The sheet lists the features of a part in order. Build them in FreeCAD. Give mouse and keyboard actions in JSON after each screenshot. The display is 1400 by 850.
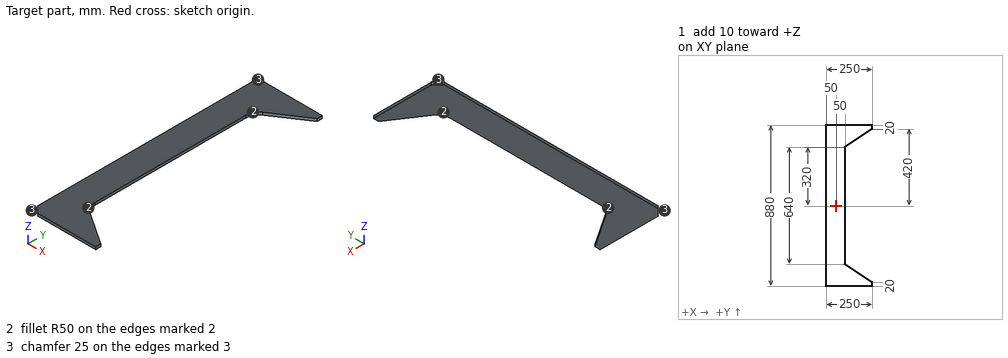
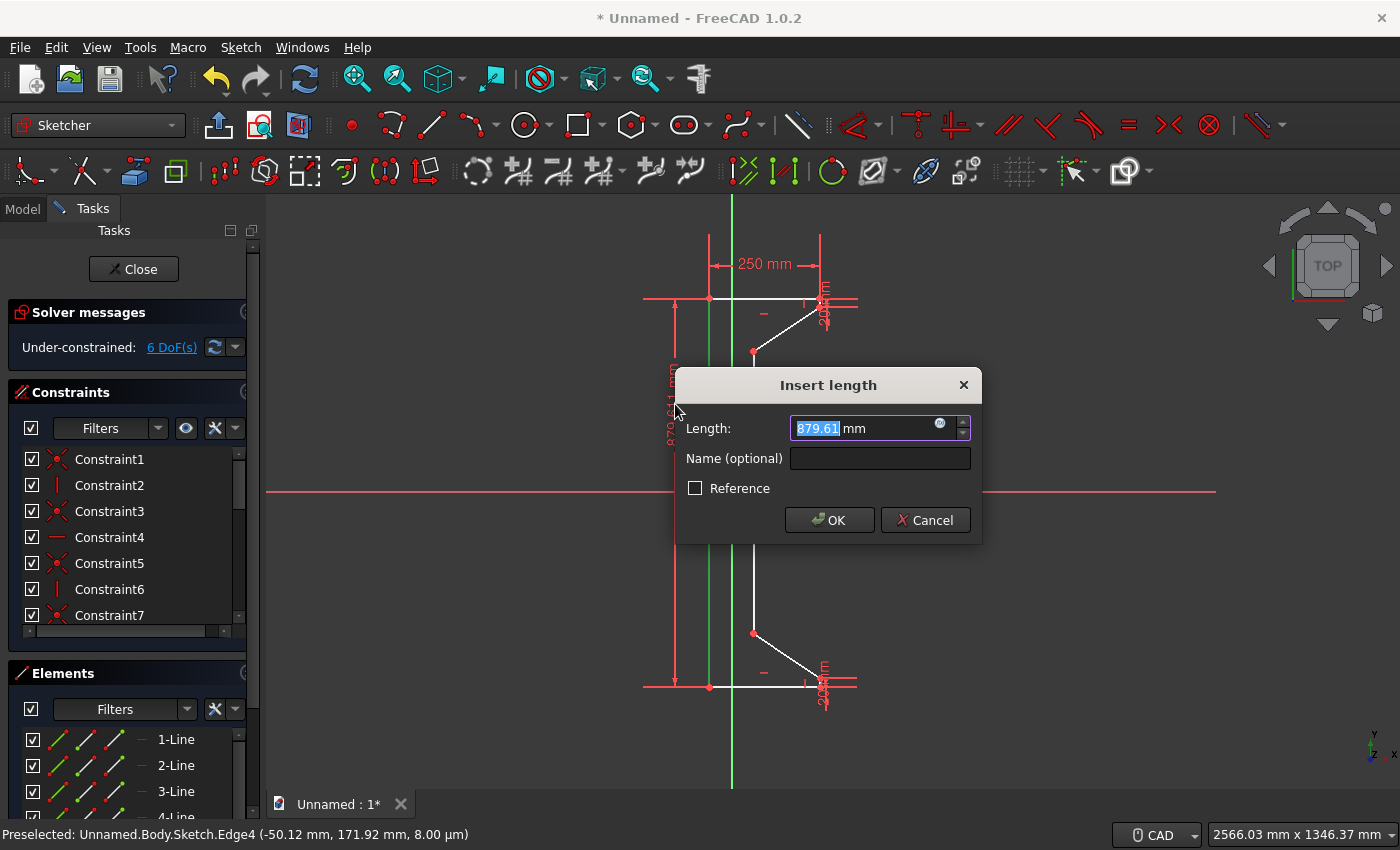
{"action": "type", "text": "880"}
{"action": "key", "text": "Return"}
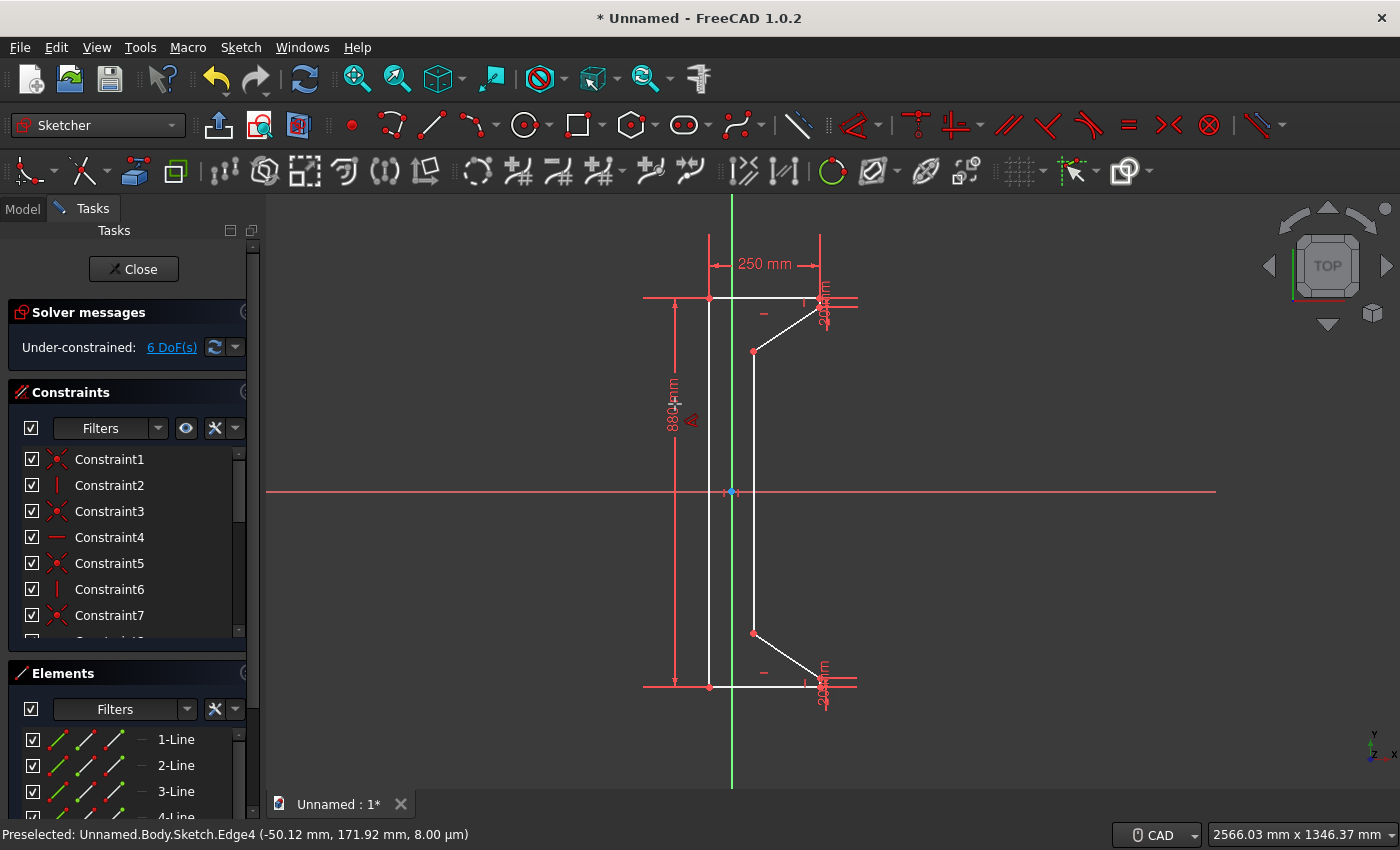
{"action": "scroll", "coordinate": [743, 687], "scroll_direction": "up", "scroll_amount": 2}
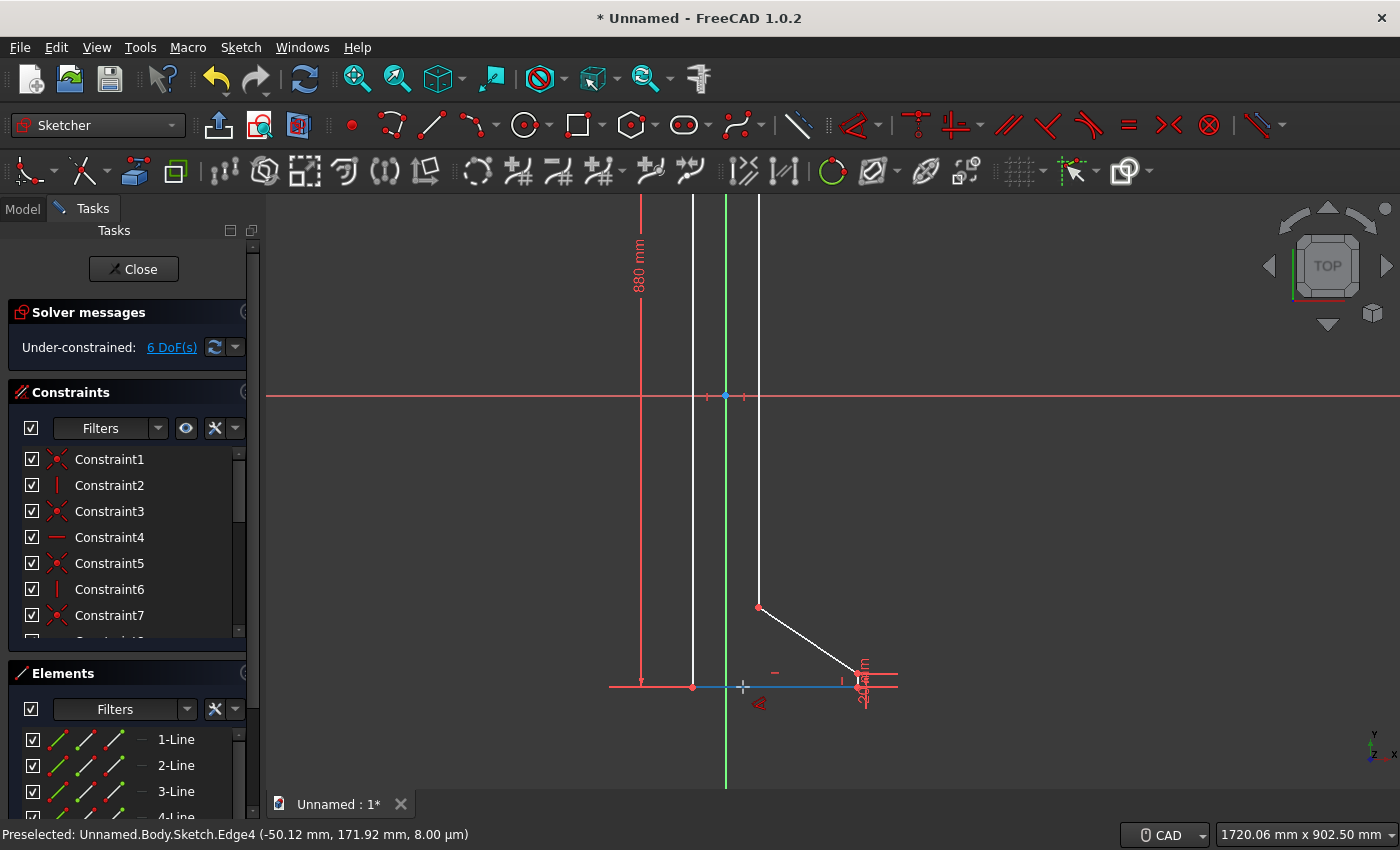
{"action": "left_click", "coordinate": [742, 687]}
{"action": "left_click", "coordinate": [775, 721]}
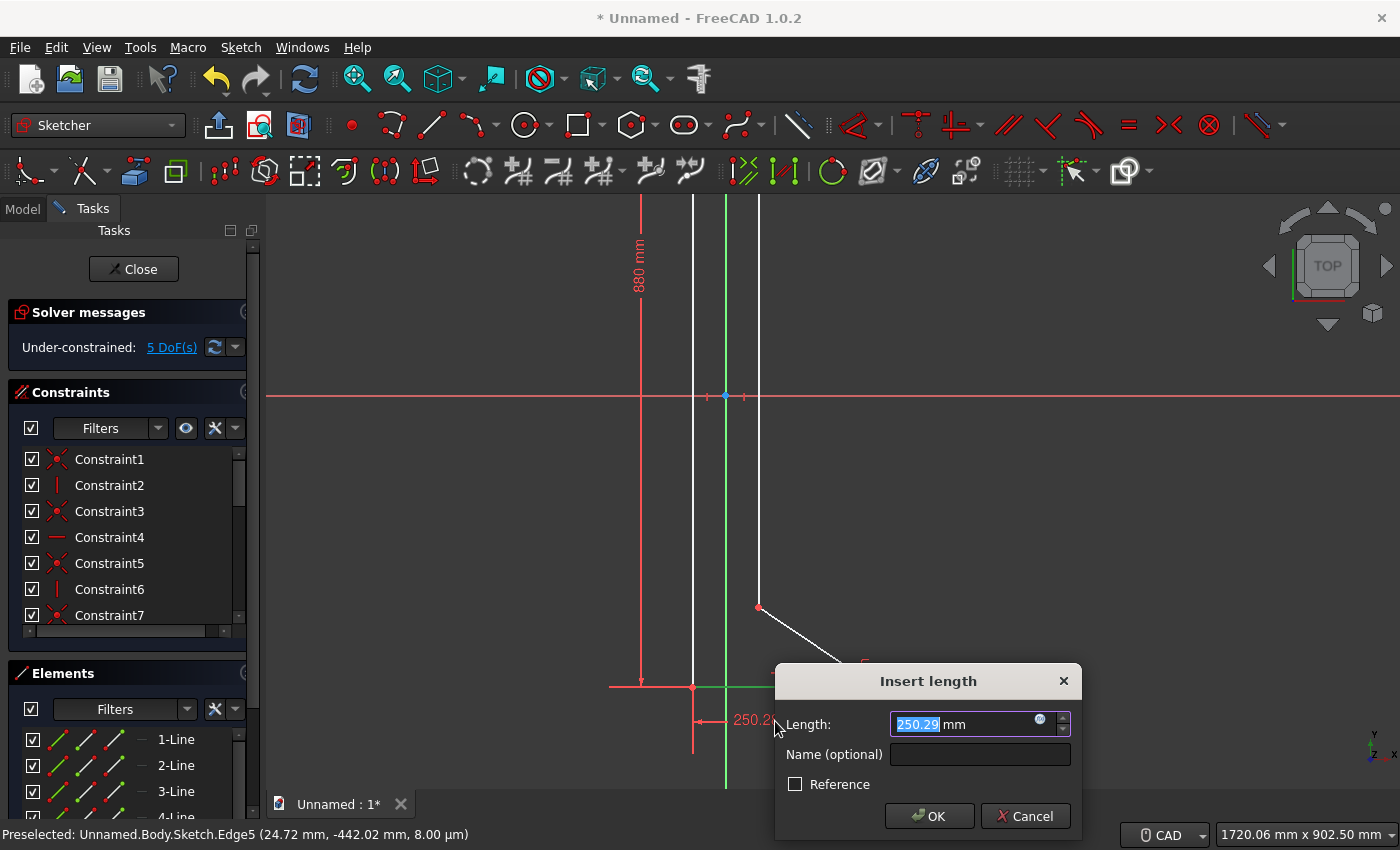
{"action": "type", "text": "250"}
{"action": "key", "text": "Return"}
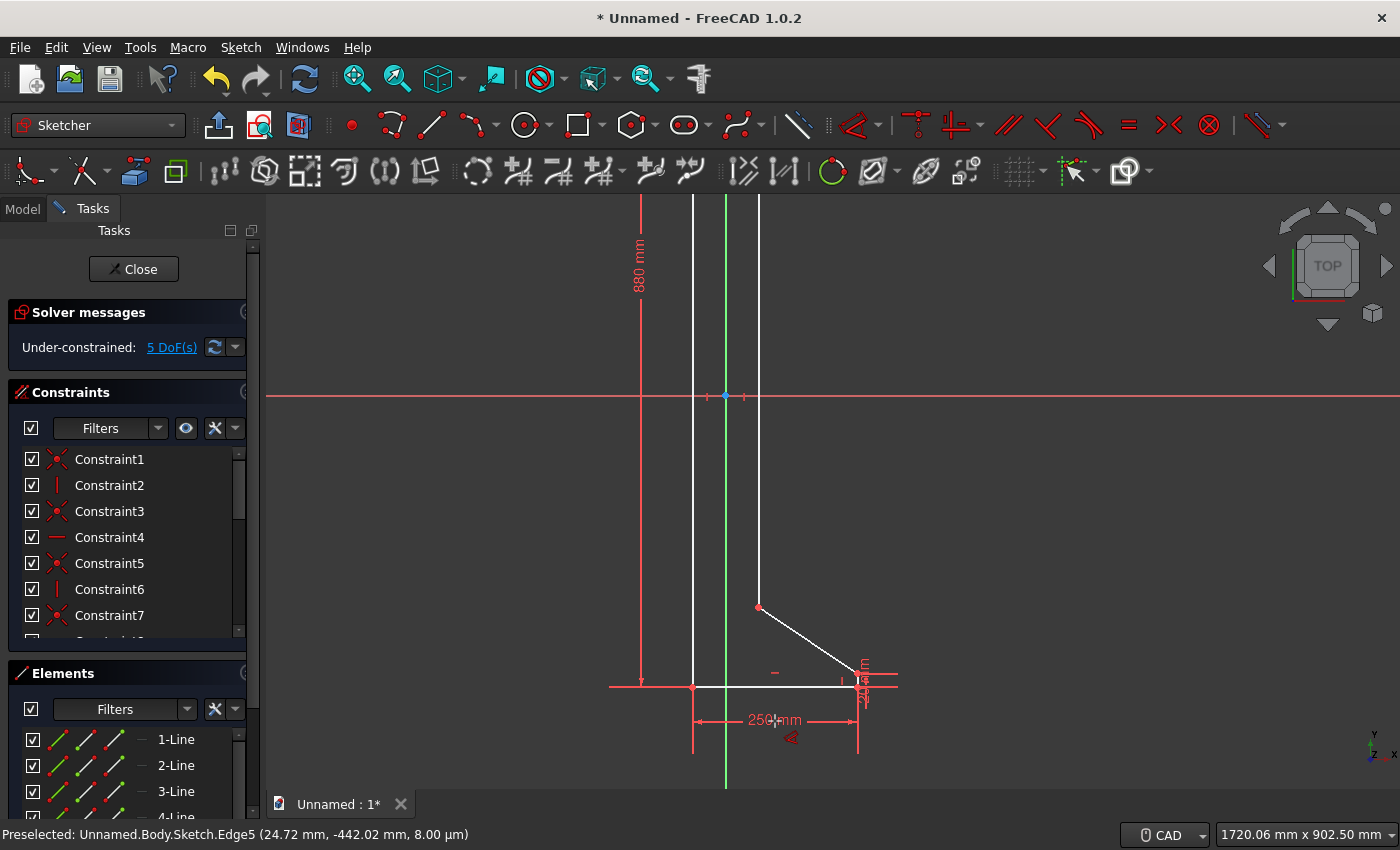
{"action": "left_click", "coordinate": [759, 481]}
{"action": "left_click", "coordinate": [793, 415]}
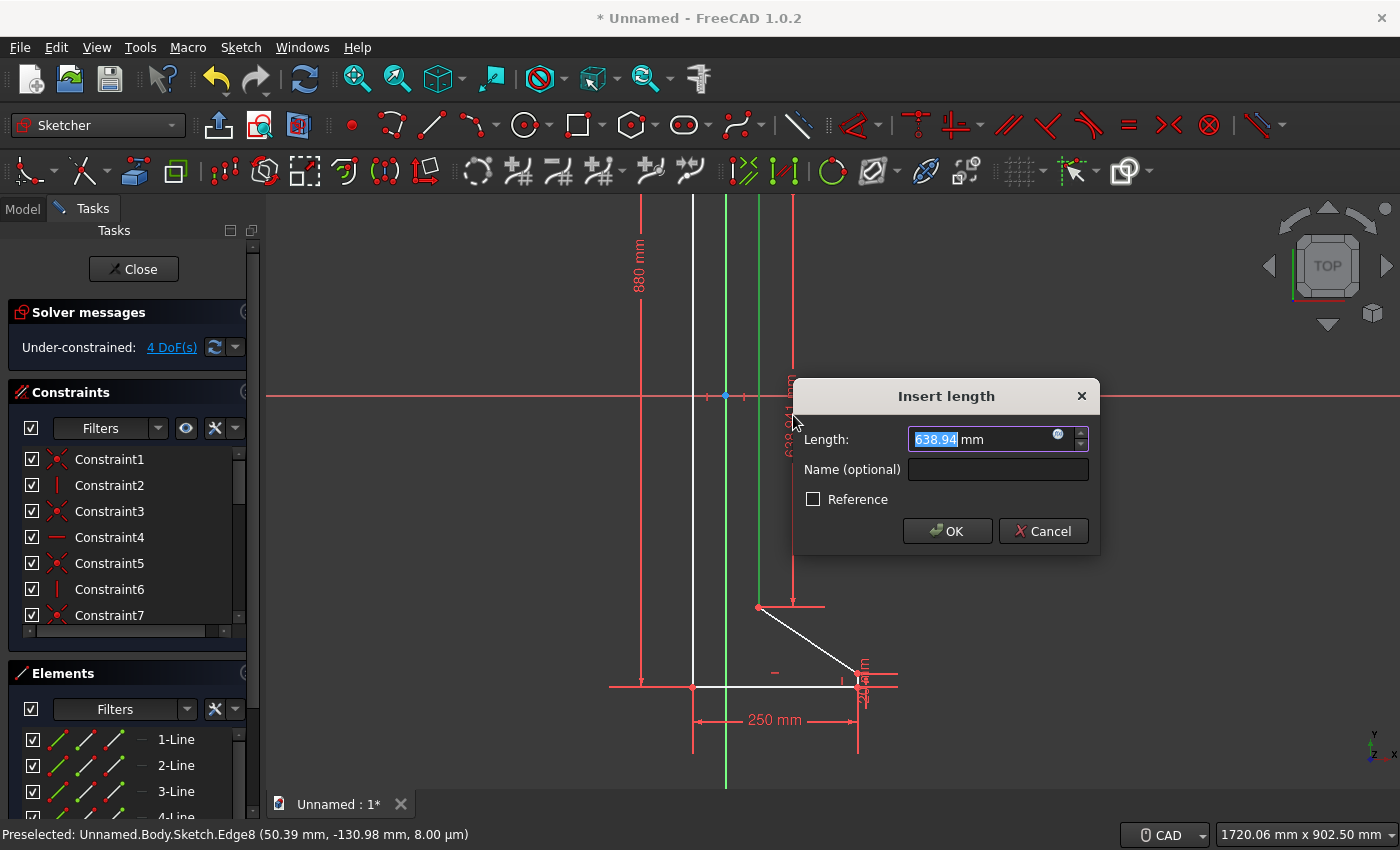
{"action": "type", "text": "640"}
{"action": "key", "text": "Return"}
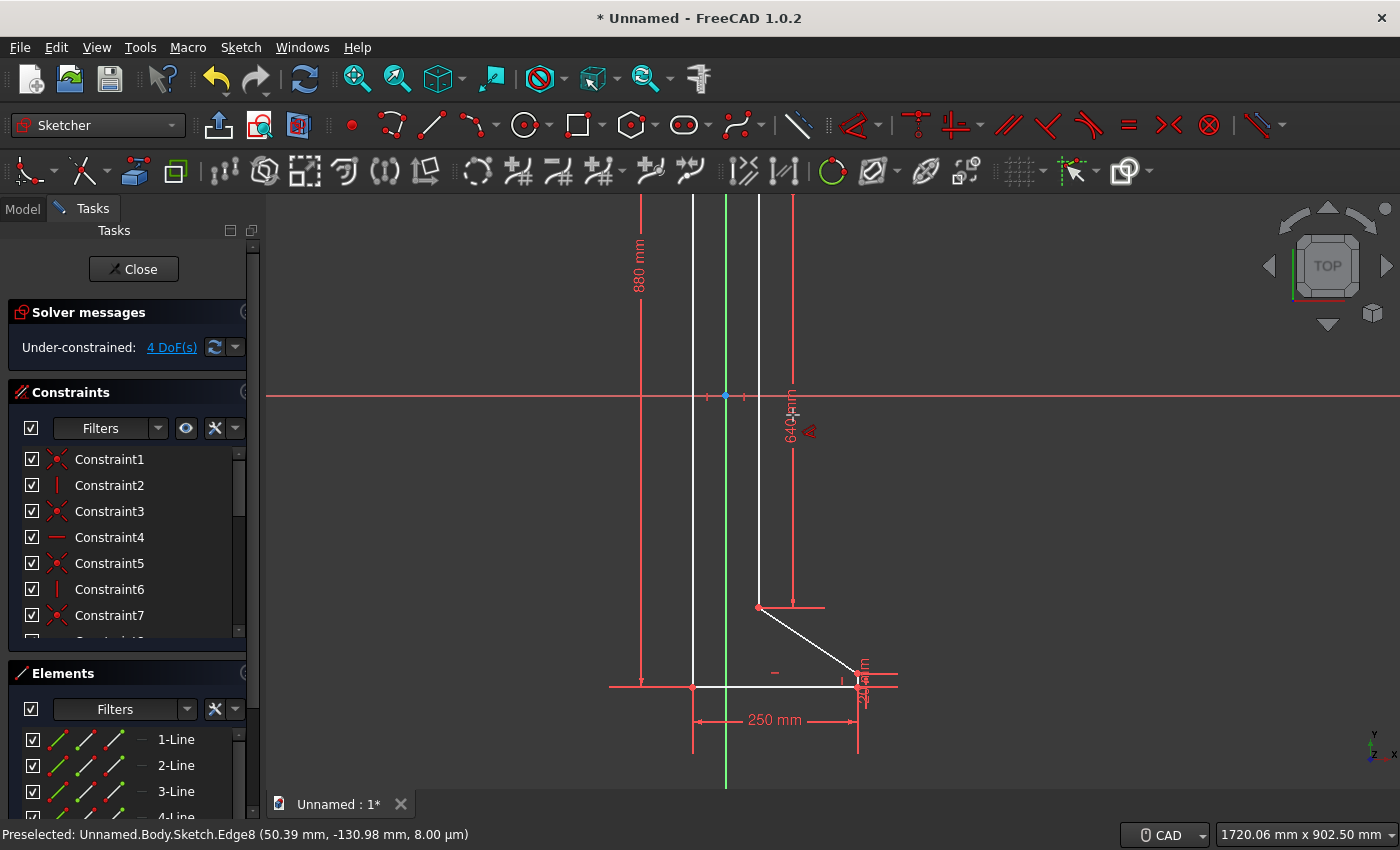
{"action": "scroll", "coordinate": [743, 686], "scroll_direction": "down", "scroll_amount": 2}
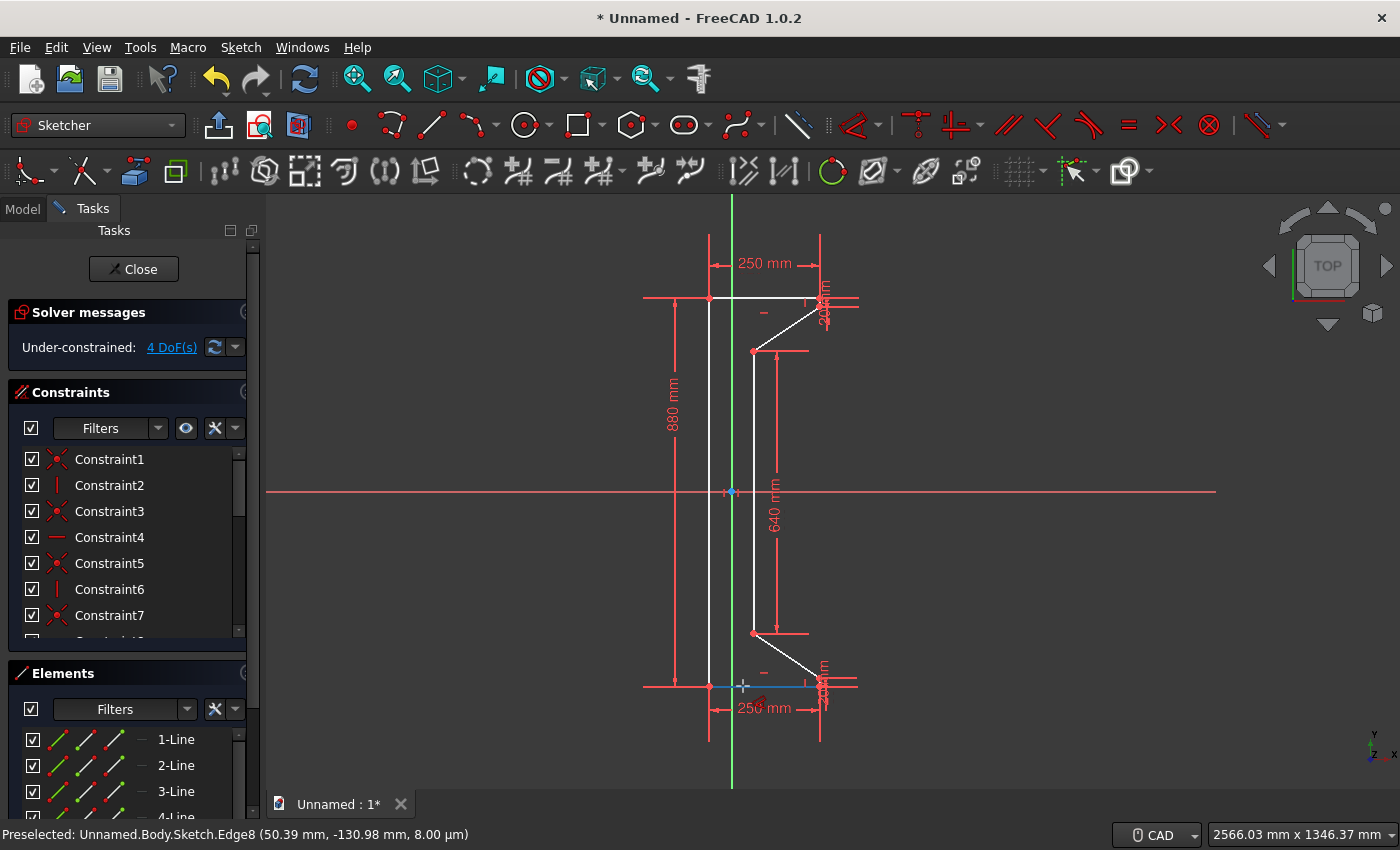
{"action": "scroll", "coordinate": [754, 351], "scroll_direction": "up", "scroll_amount": 3}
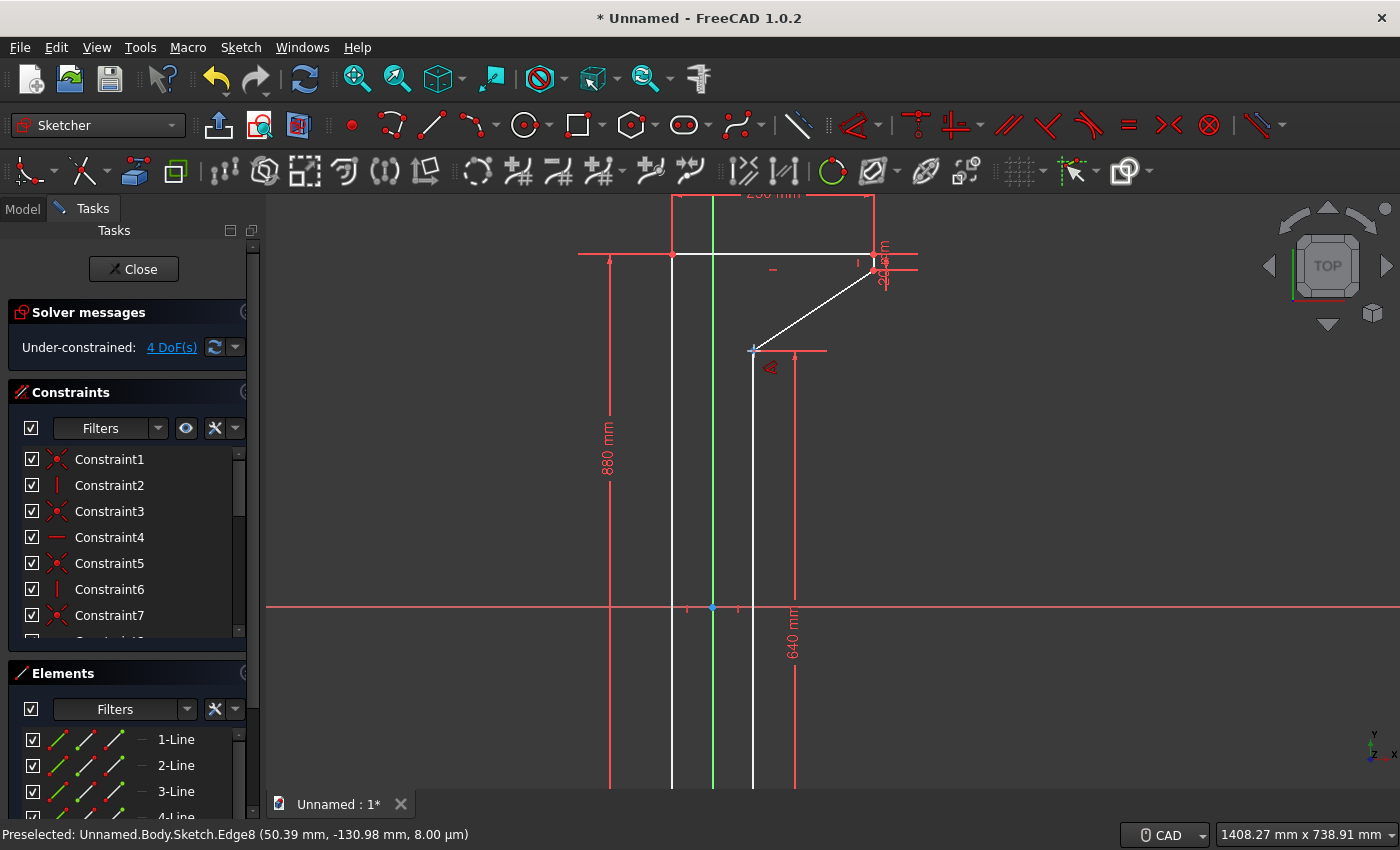
{"action": "left_click", "coordinate": [753, 351]}
{"action": "left_click", "coordinate": [733, 317]}